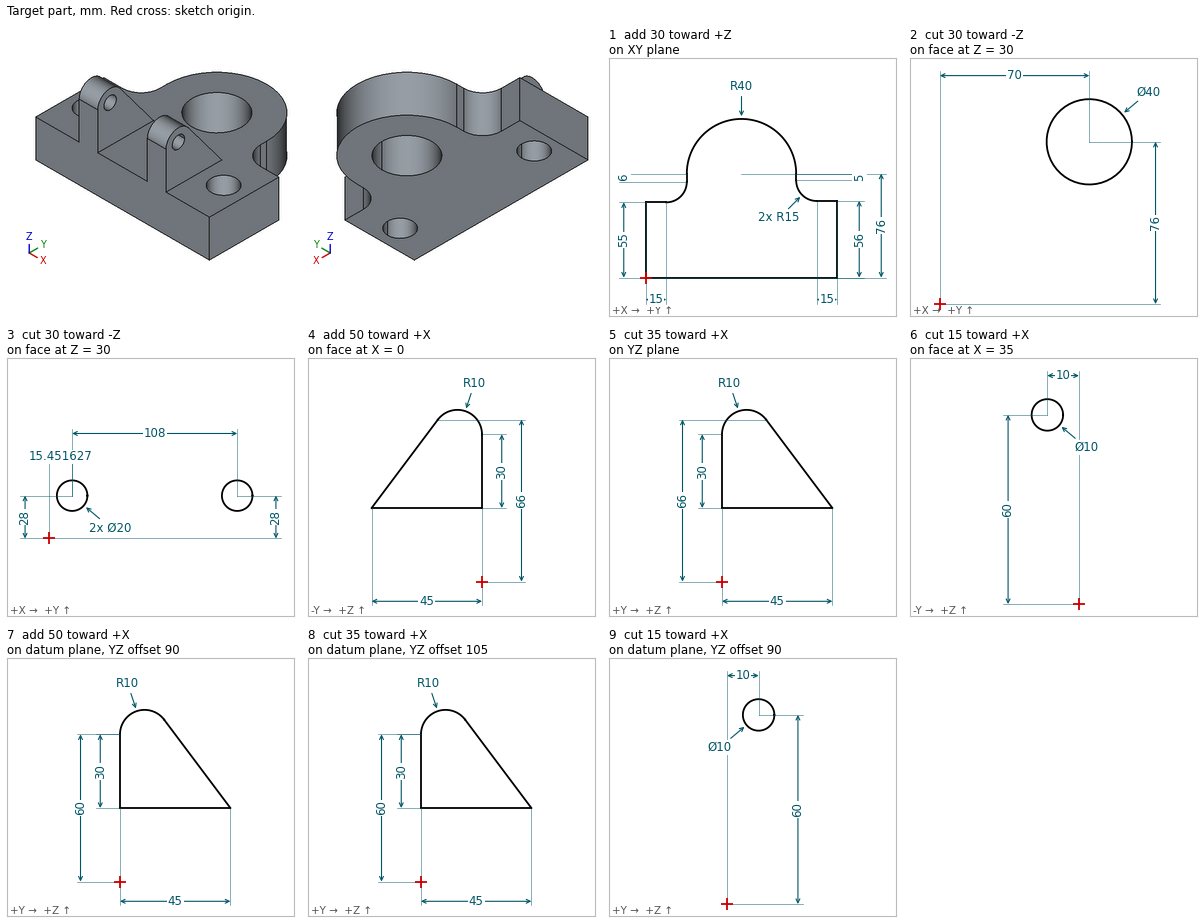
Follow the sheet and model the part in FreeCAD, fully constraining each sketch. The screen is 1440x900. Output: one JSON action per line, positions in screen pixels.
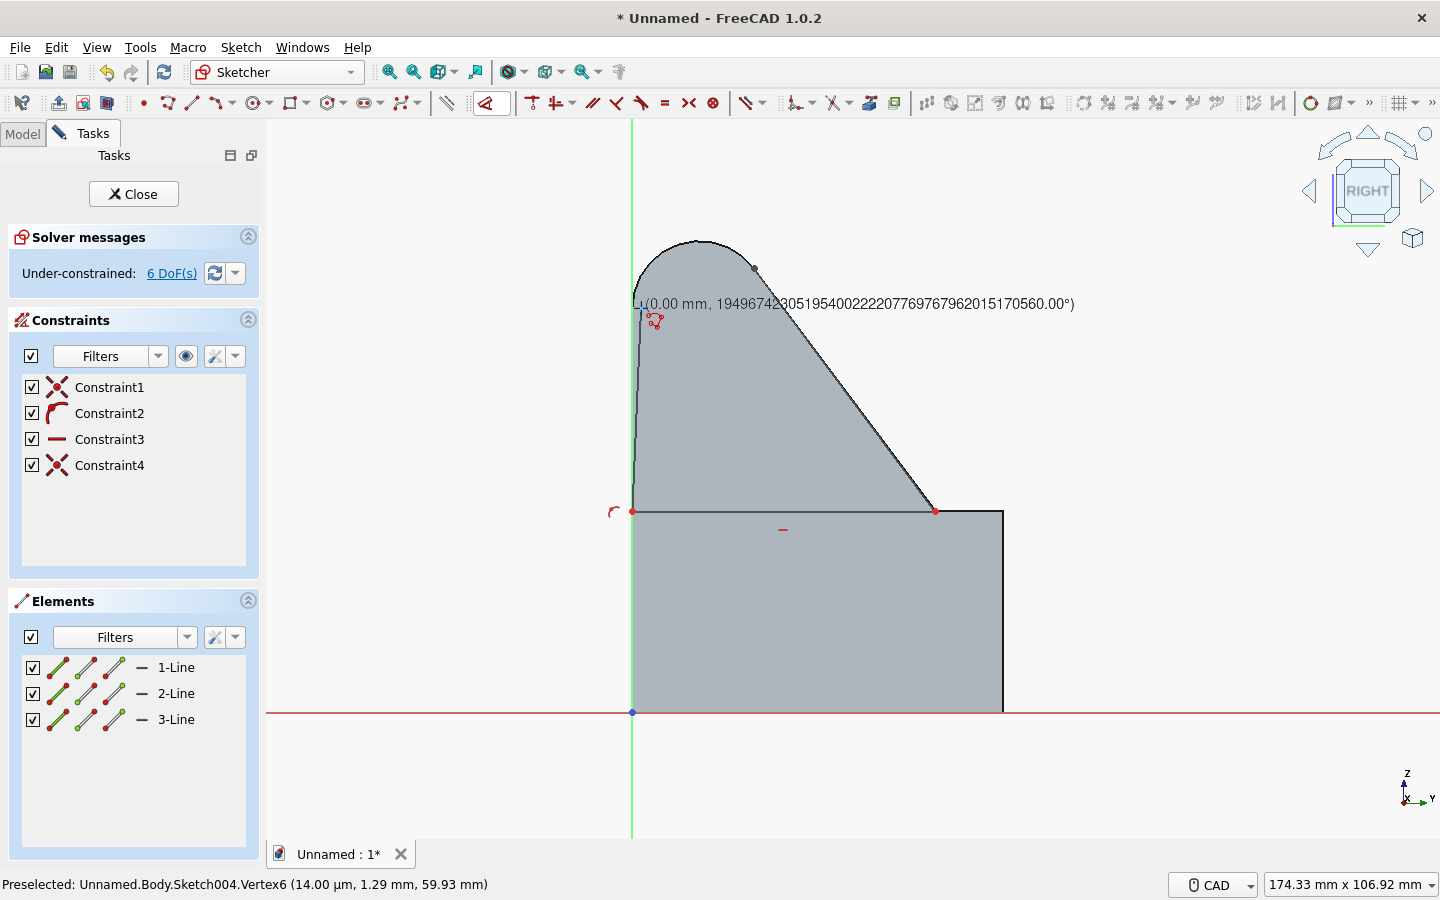
{"action": "key", "text": "g 3 a"}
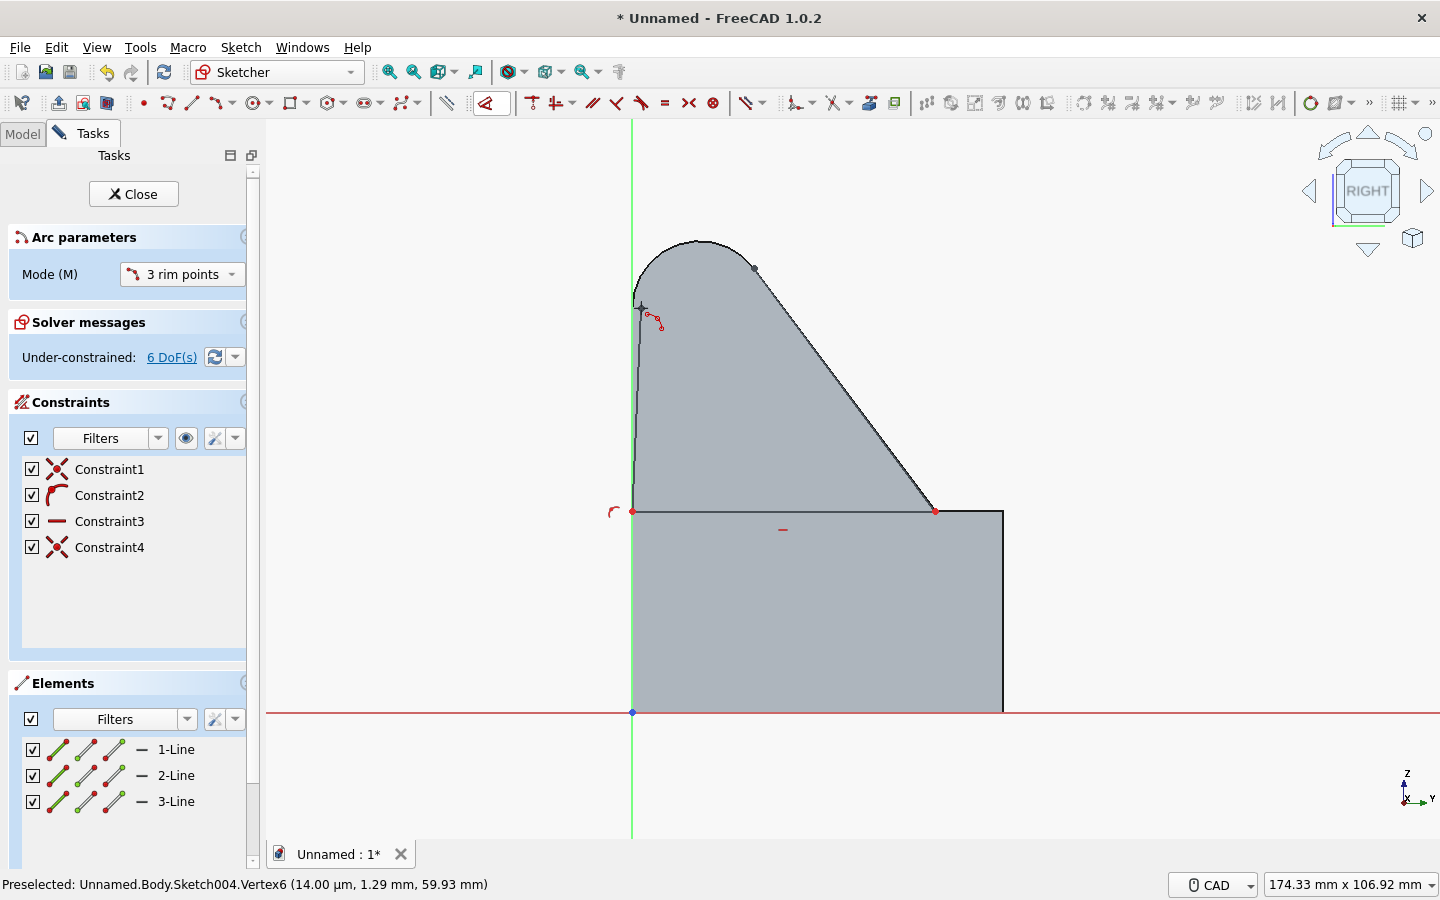
{"action": "left_click", "coordinate": [641, 309]}
{"action": "left_click", "coordinate": [754, 269]}
{"action": "left_click", "coordinate": [678, 245]}
{"action": "key", "text": "Escape"}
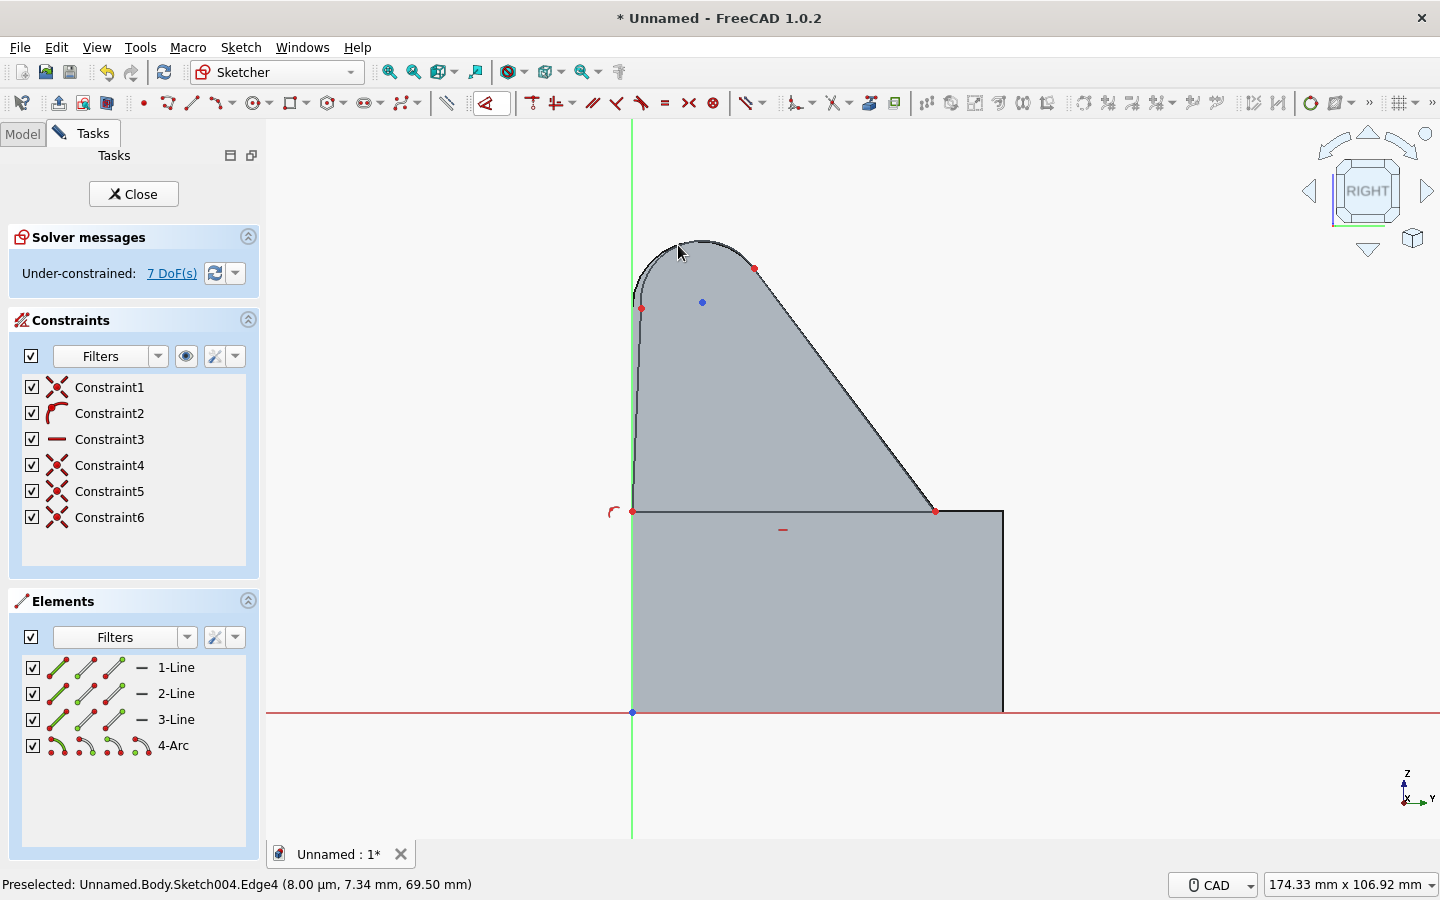
{"action": "left_click", "coordinate": [808, 342]}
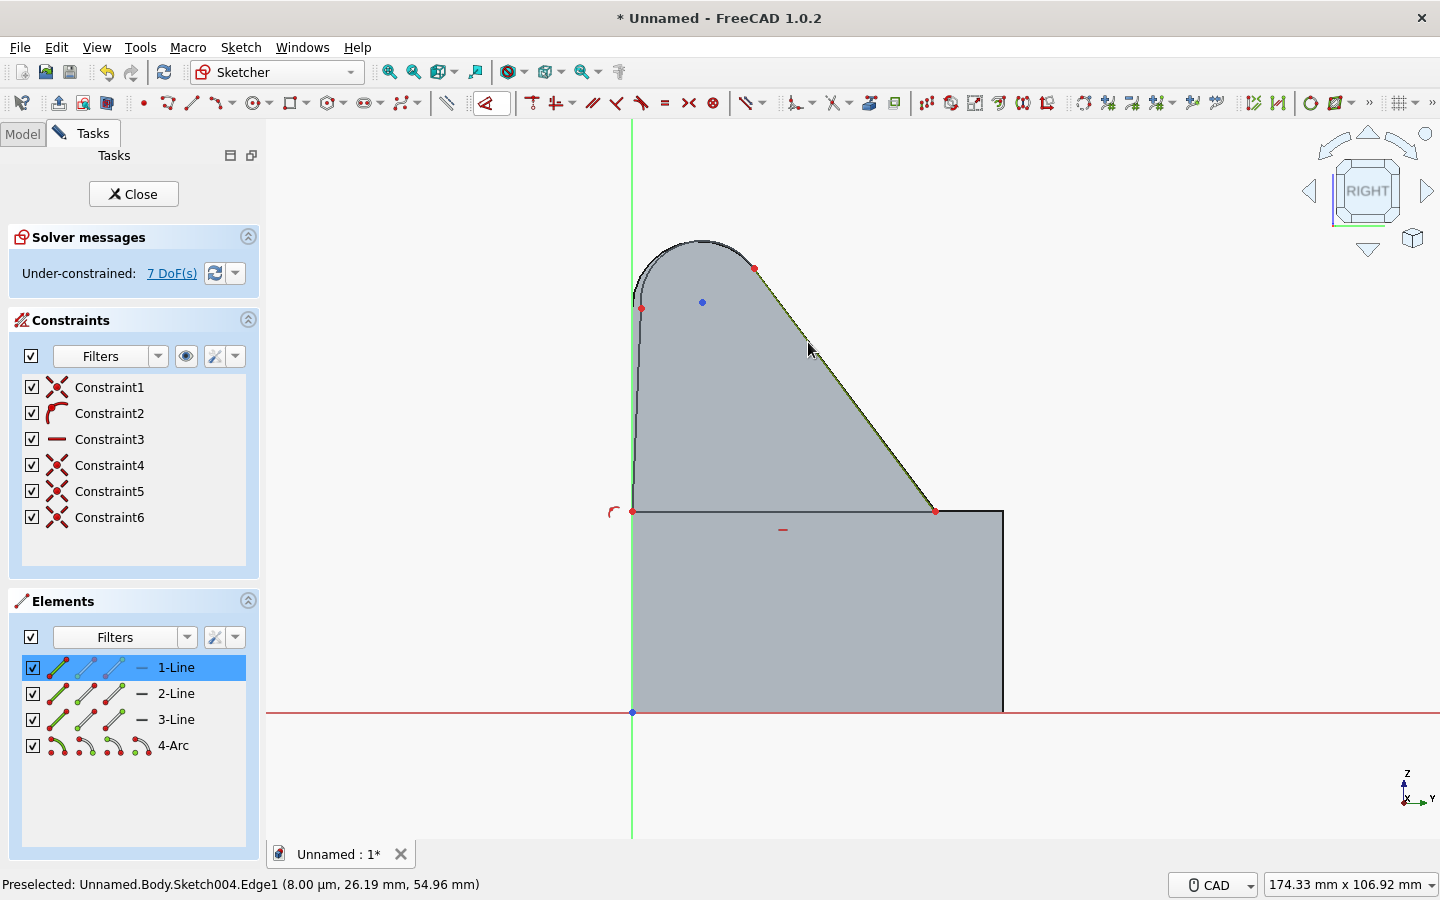
{"action": "left_click", "coordinate": [714, 242]}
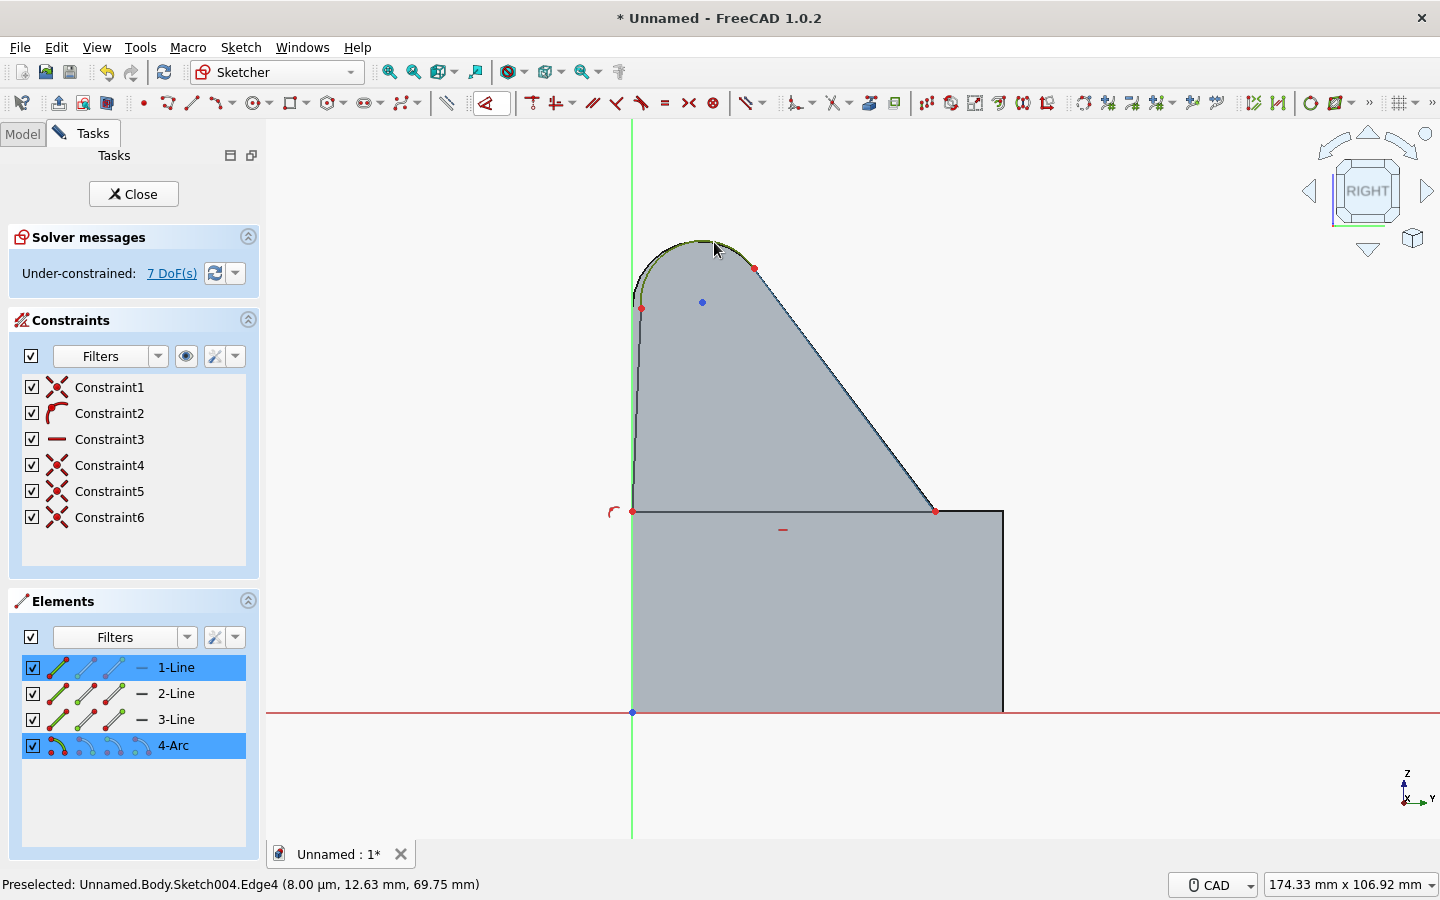
{"action": "left_click", "coordinate": [642, 104]}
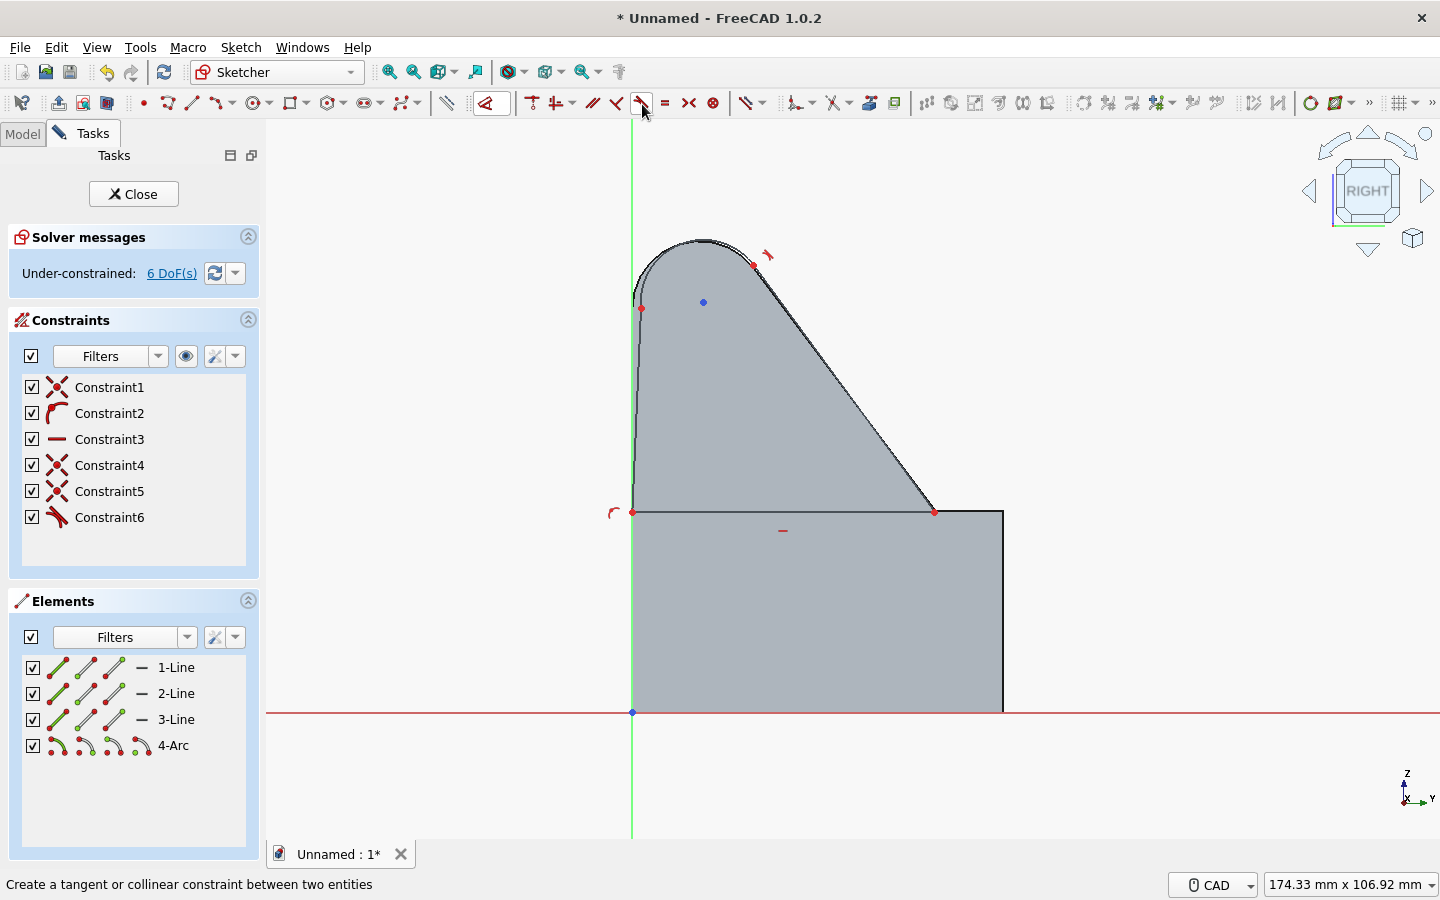
{"action": "left_click", "coordinate": [635, 451]}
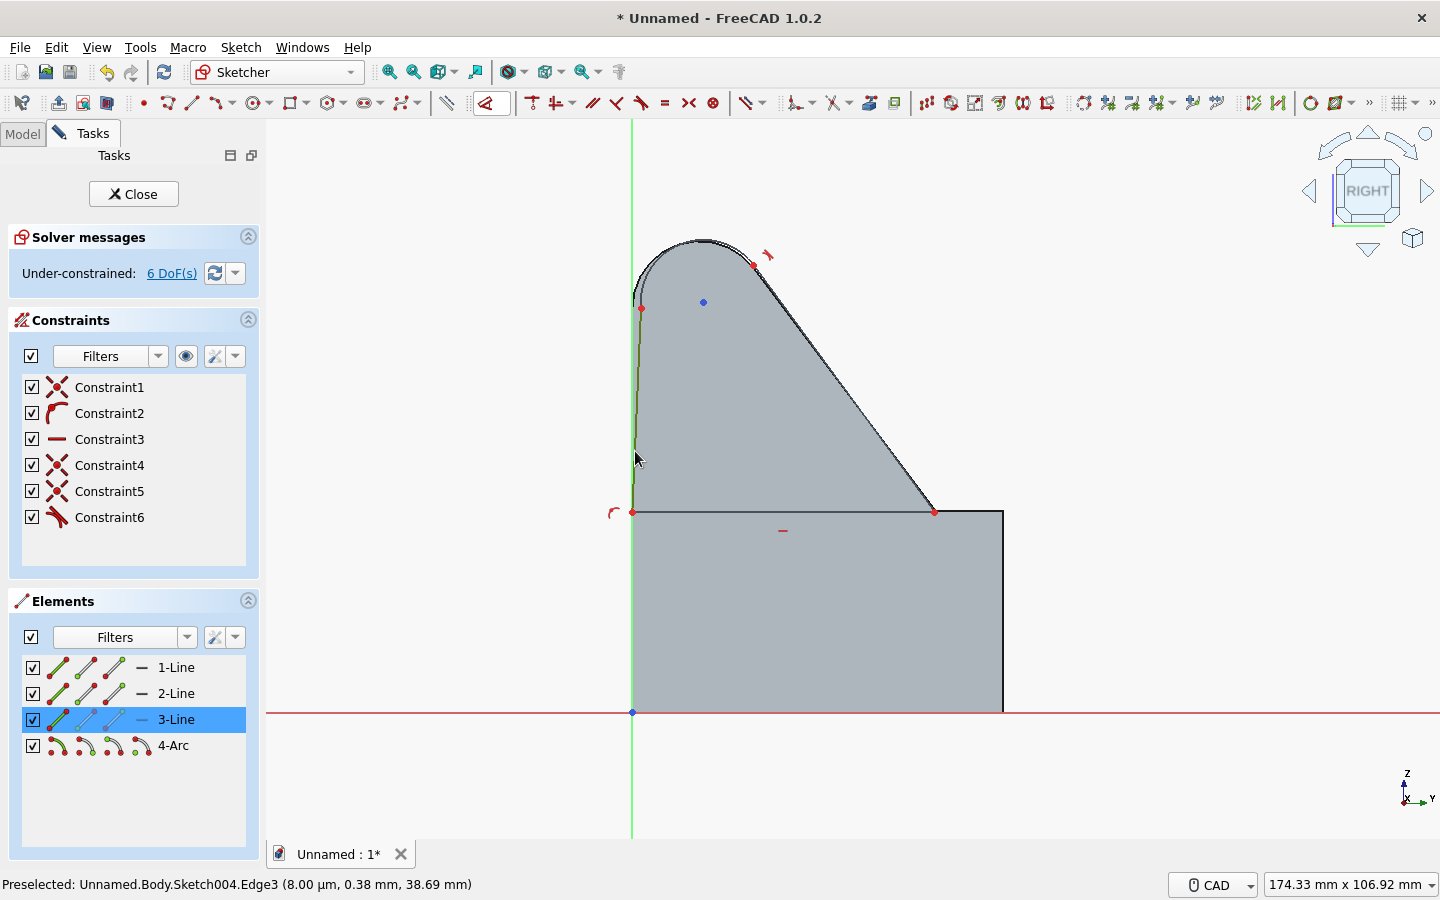
{"action": "left_click", "coordinate": [713, 241]}